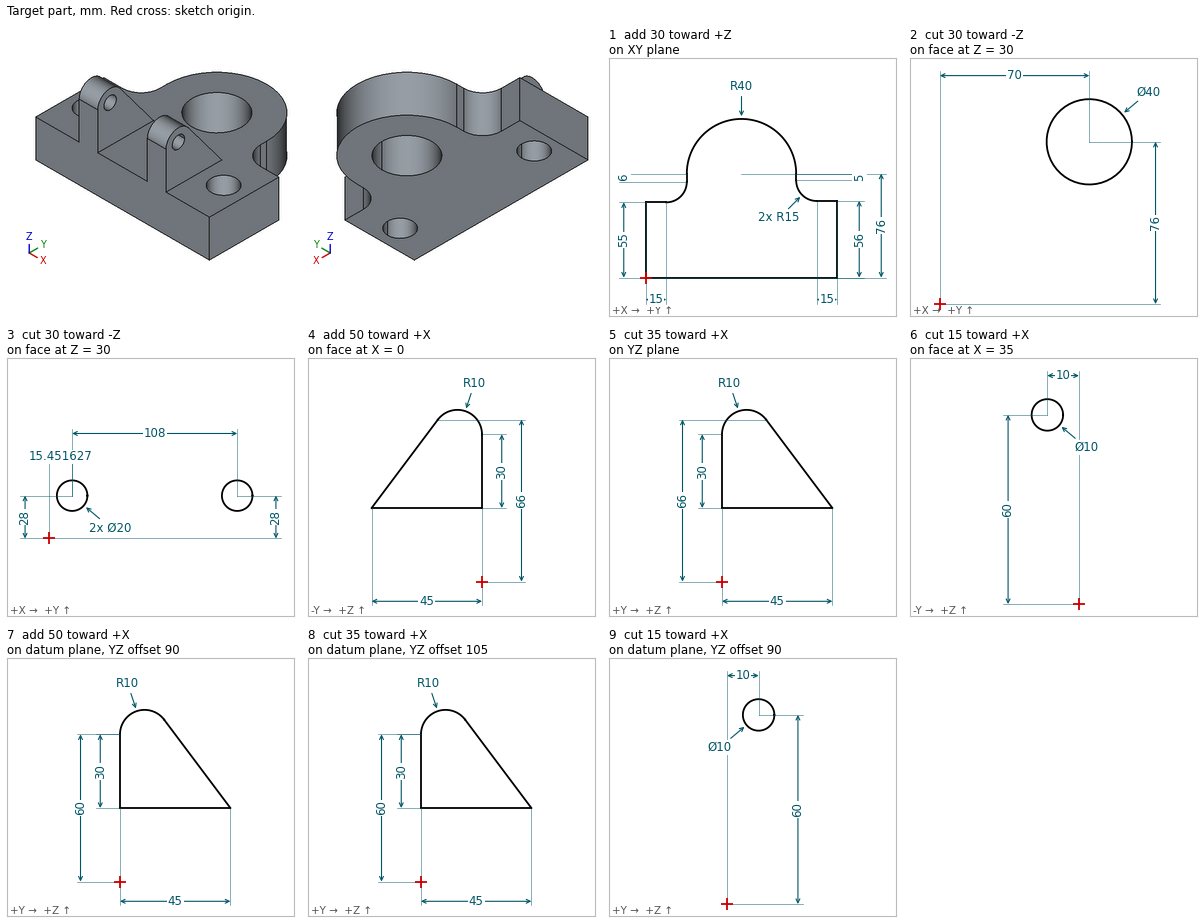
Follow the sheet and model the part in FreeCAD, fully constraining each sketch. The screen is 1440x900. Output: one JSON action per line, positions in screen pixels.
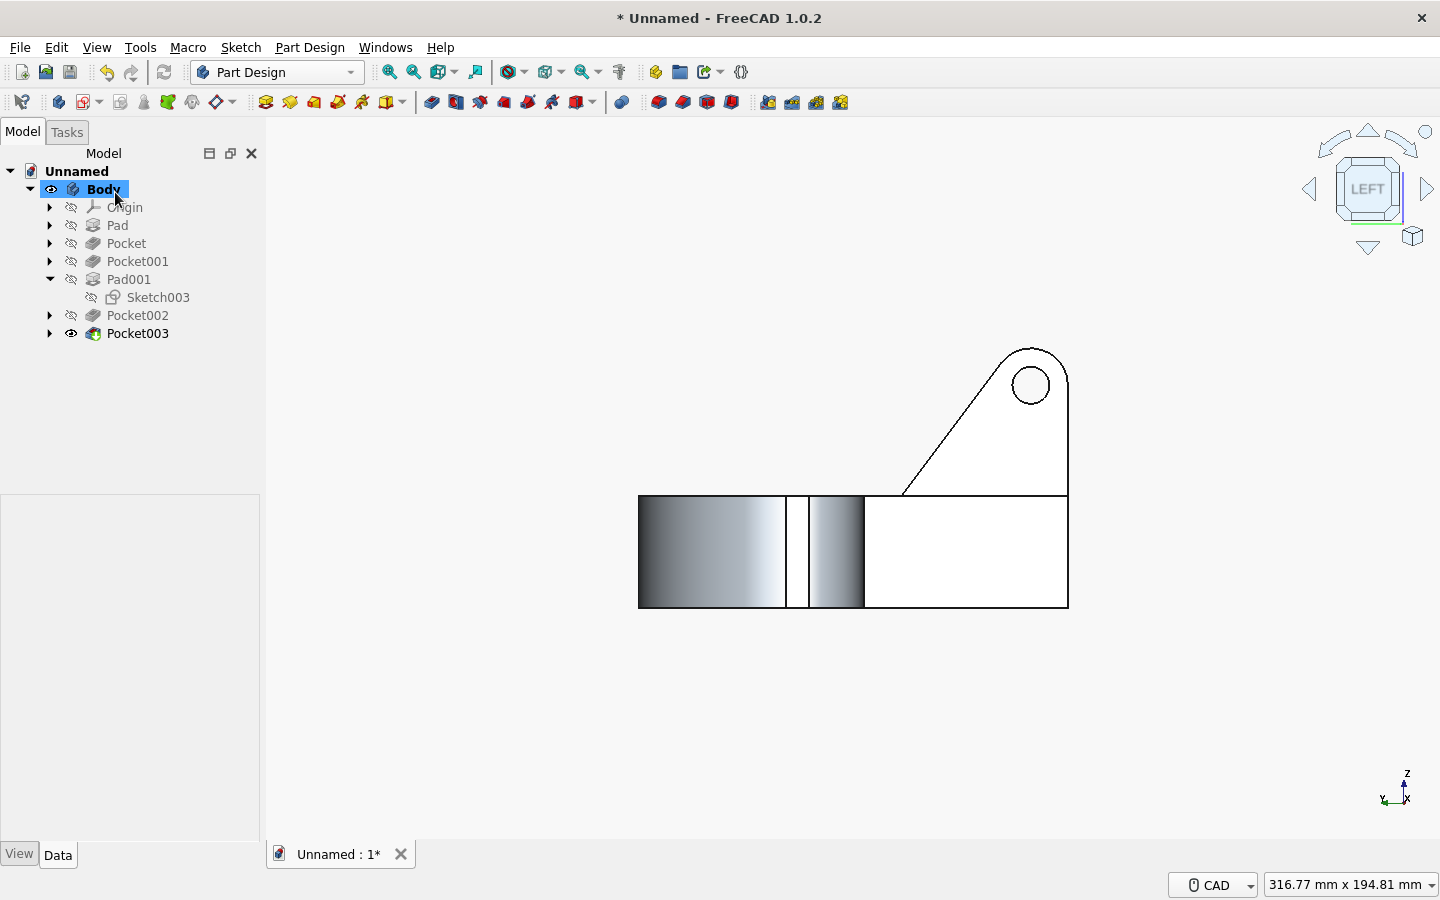
{"action": "left_click", "coordinate": [50, 207]}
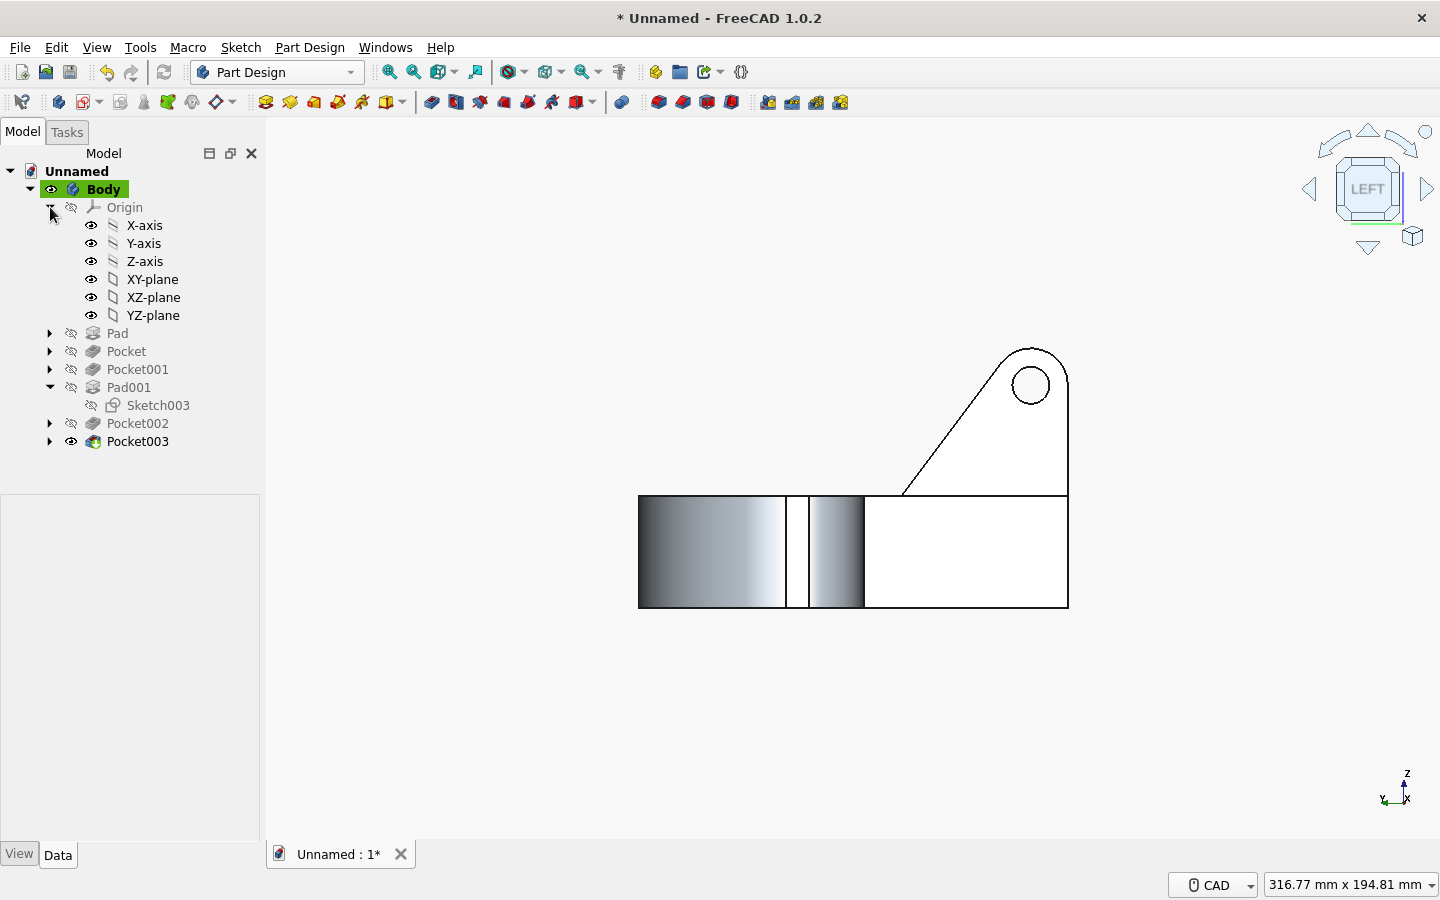
{"action": "left_click", "coordinate": [136, 315]}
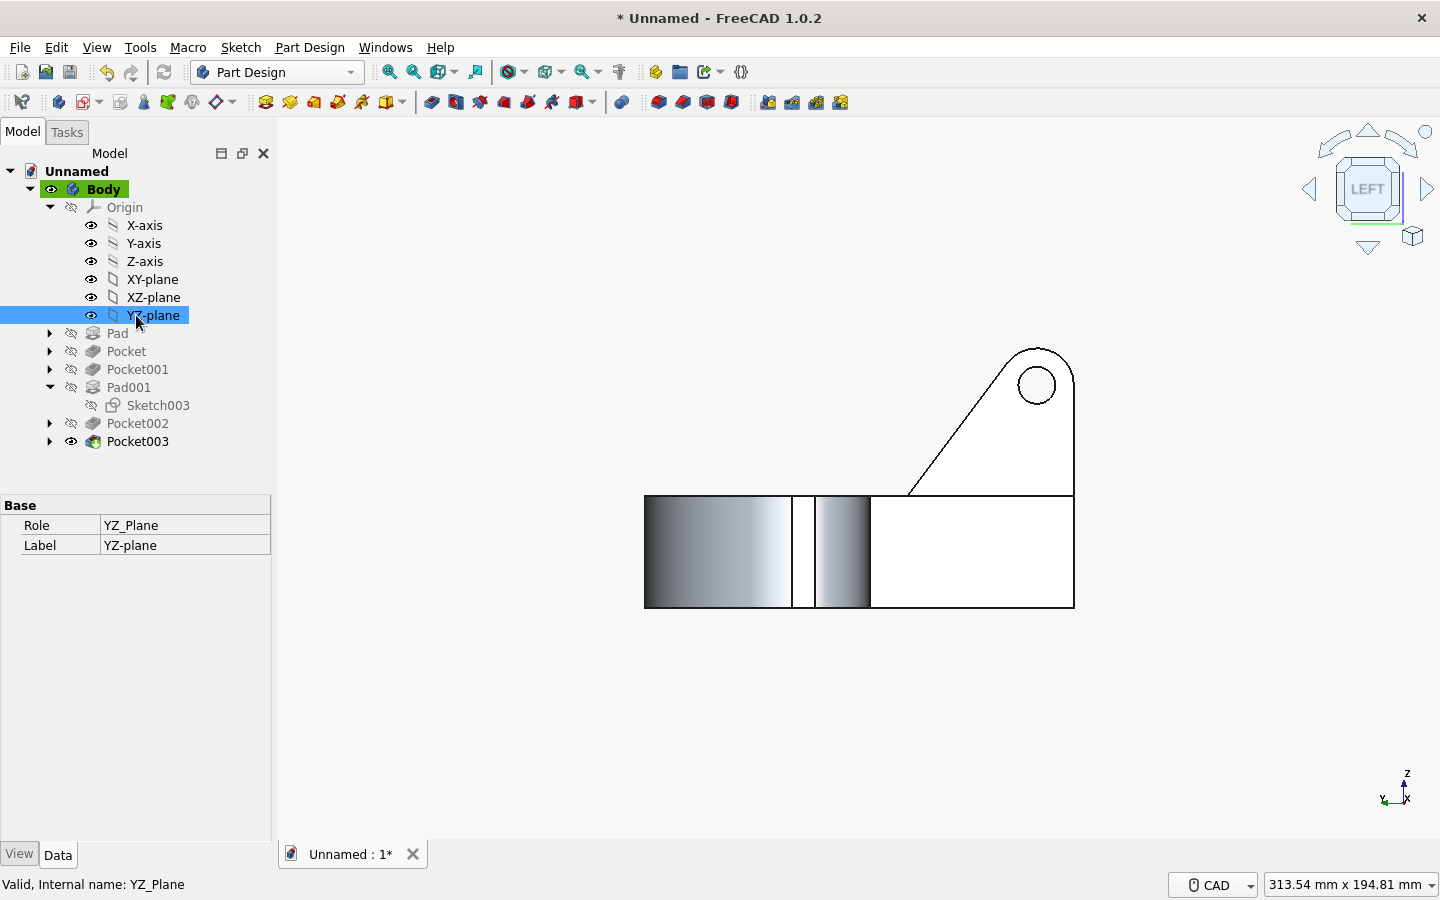
{"action": "left_click", "coordinate": [216, 102]}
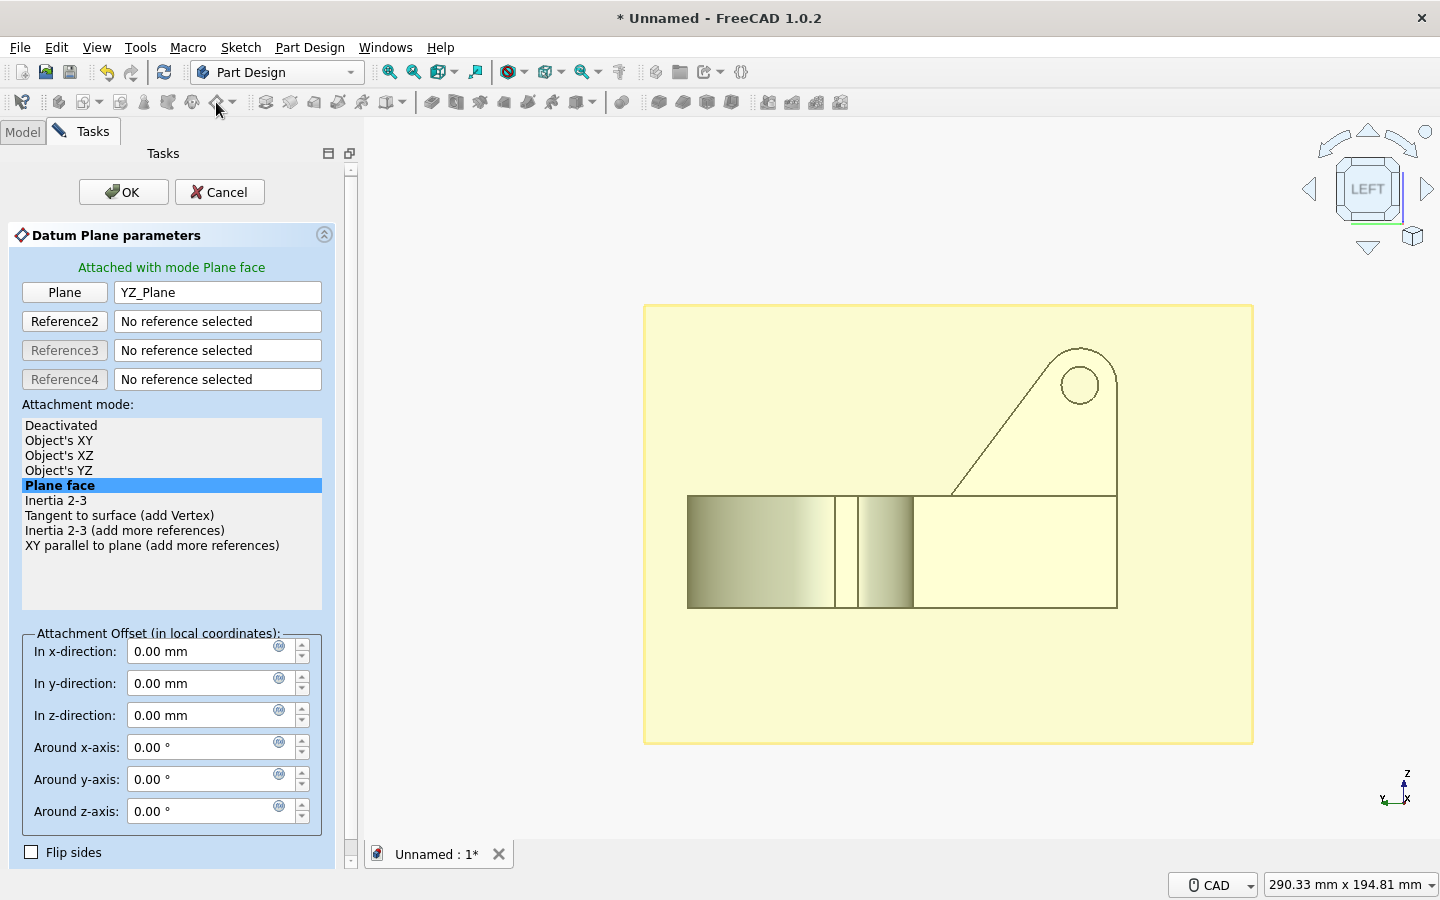
{"action": "triple_click", "coordinate": [210, 715]}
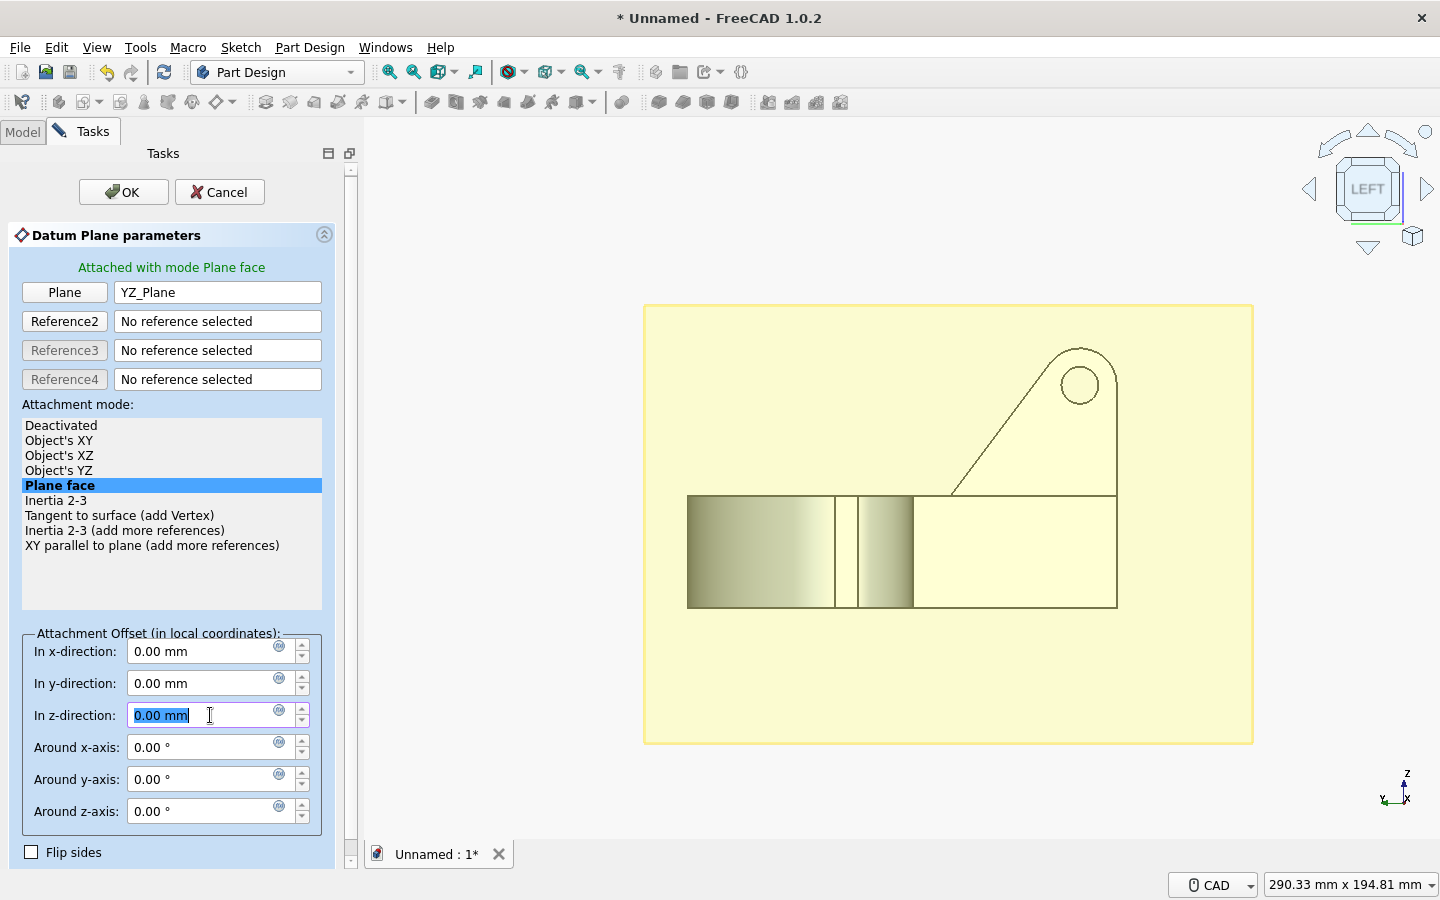
{"action": "type", "text": "90"}
{"action": "key", "text": "Tab"}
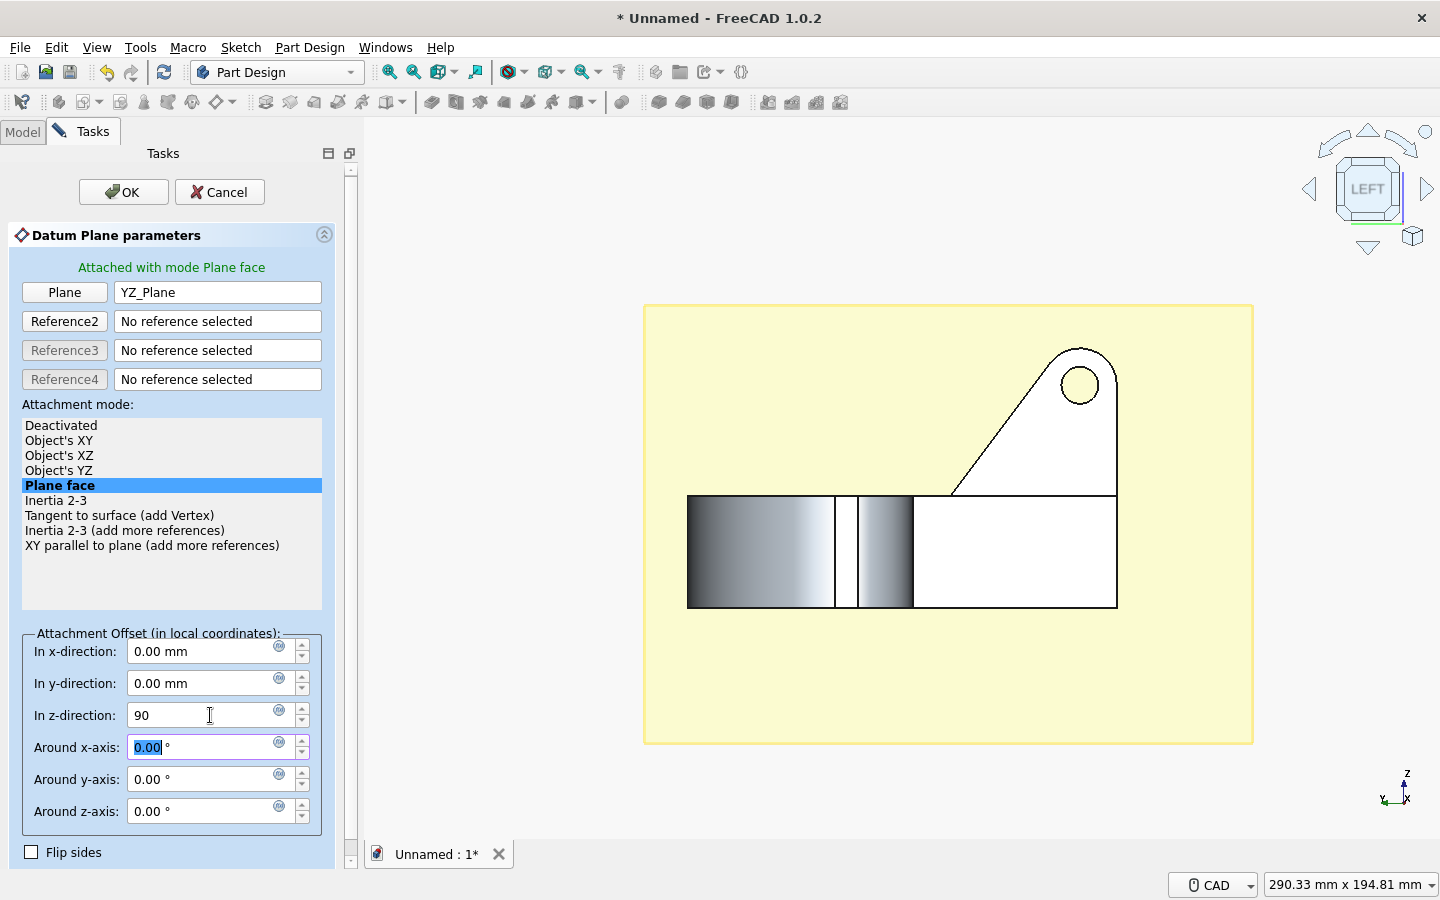
{"action": "left_click", "coordinate": [124, 192]}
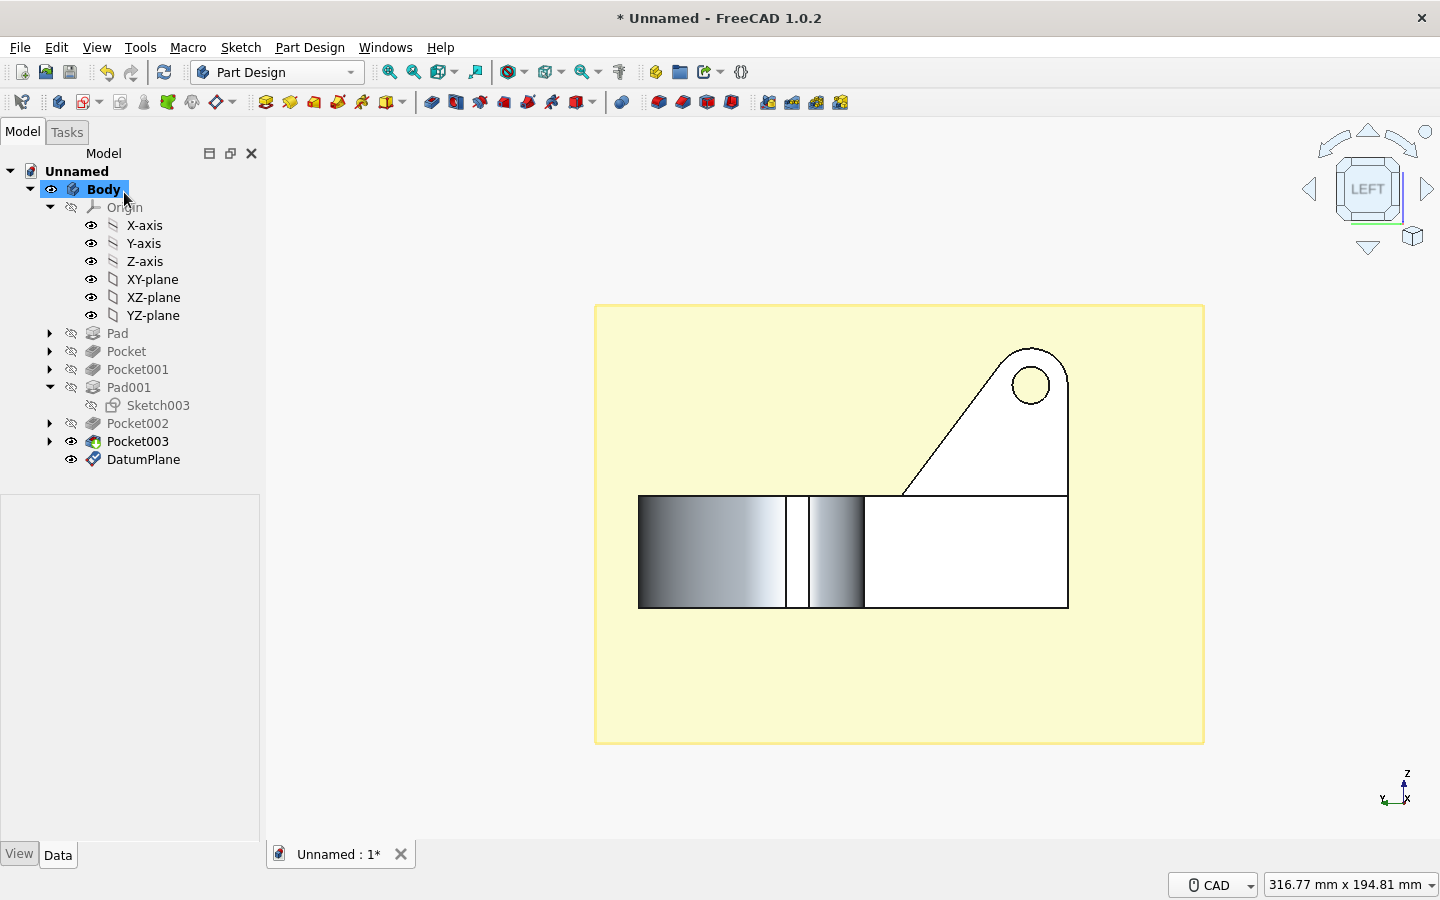
{"action": "left_click", "coordinate": [116, 459]}